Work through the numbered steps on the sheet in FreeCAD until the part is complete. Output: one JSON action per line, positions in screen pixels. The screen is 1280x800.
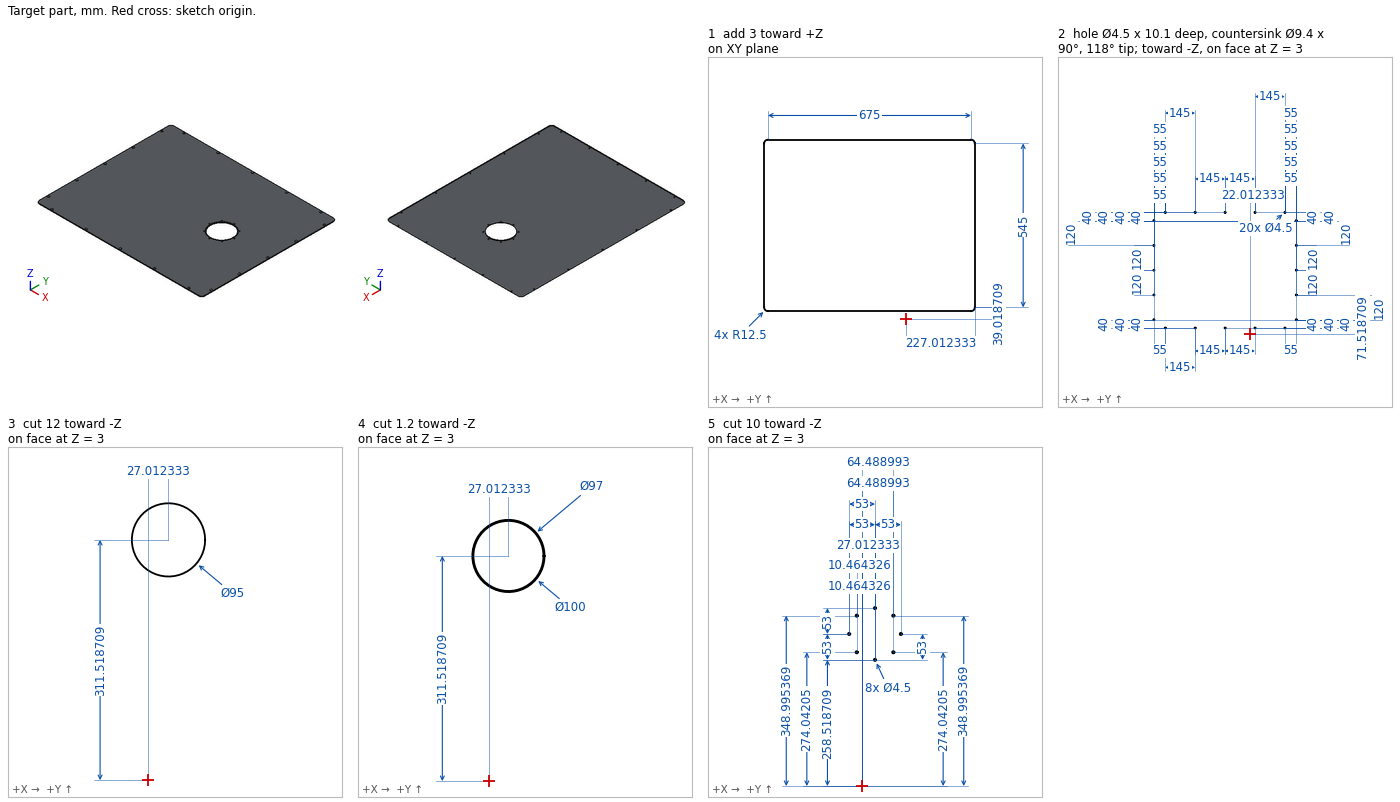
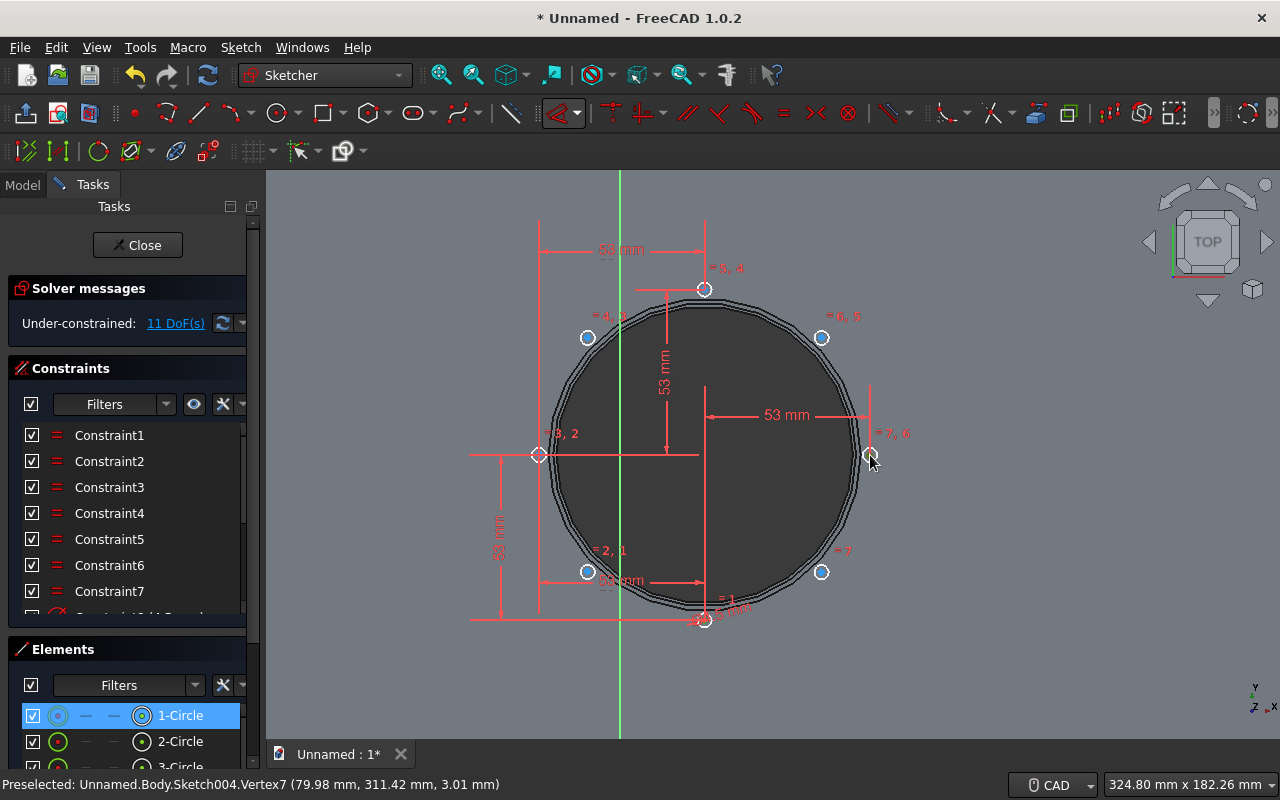
{"action": "left_click", "coordinate": [580, 114]}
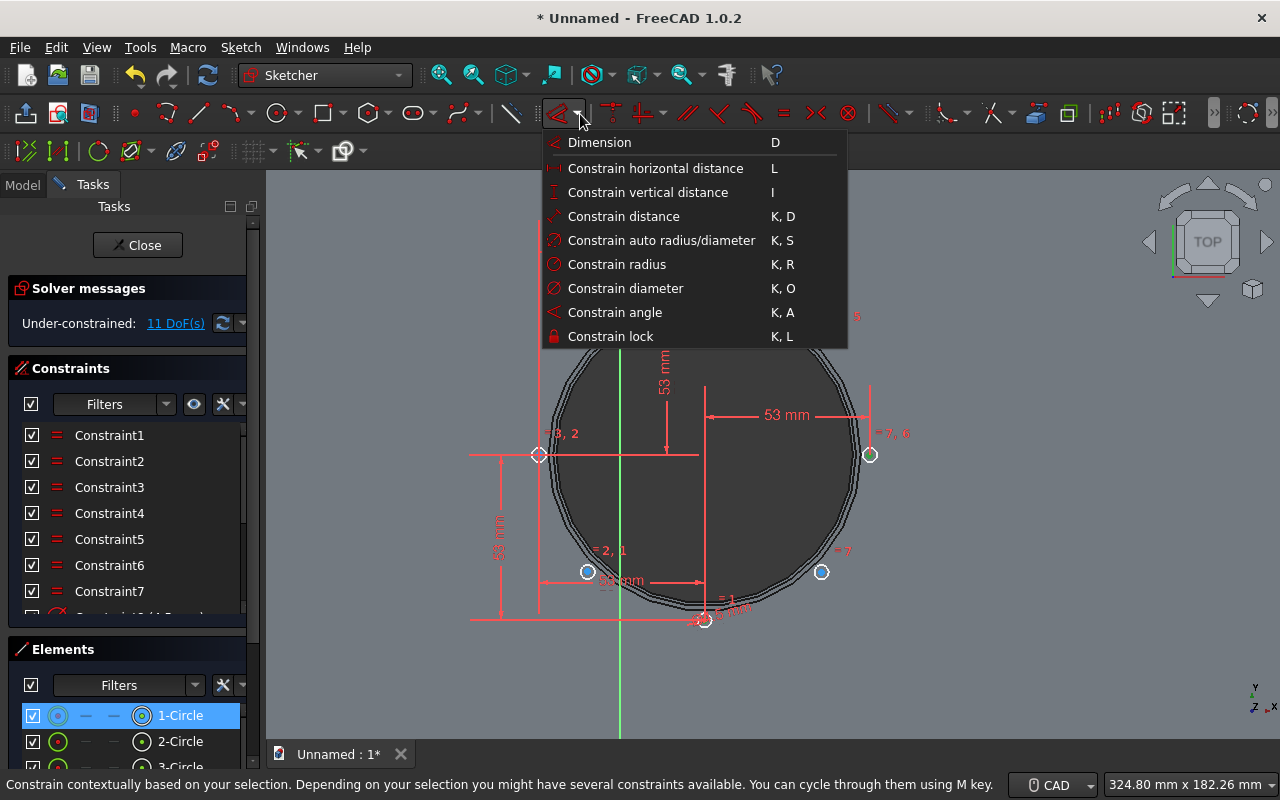
{"action": "left_click", "coordinate": [695, 192]}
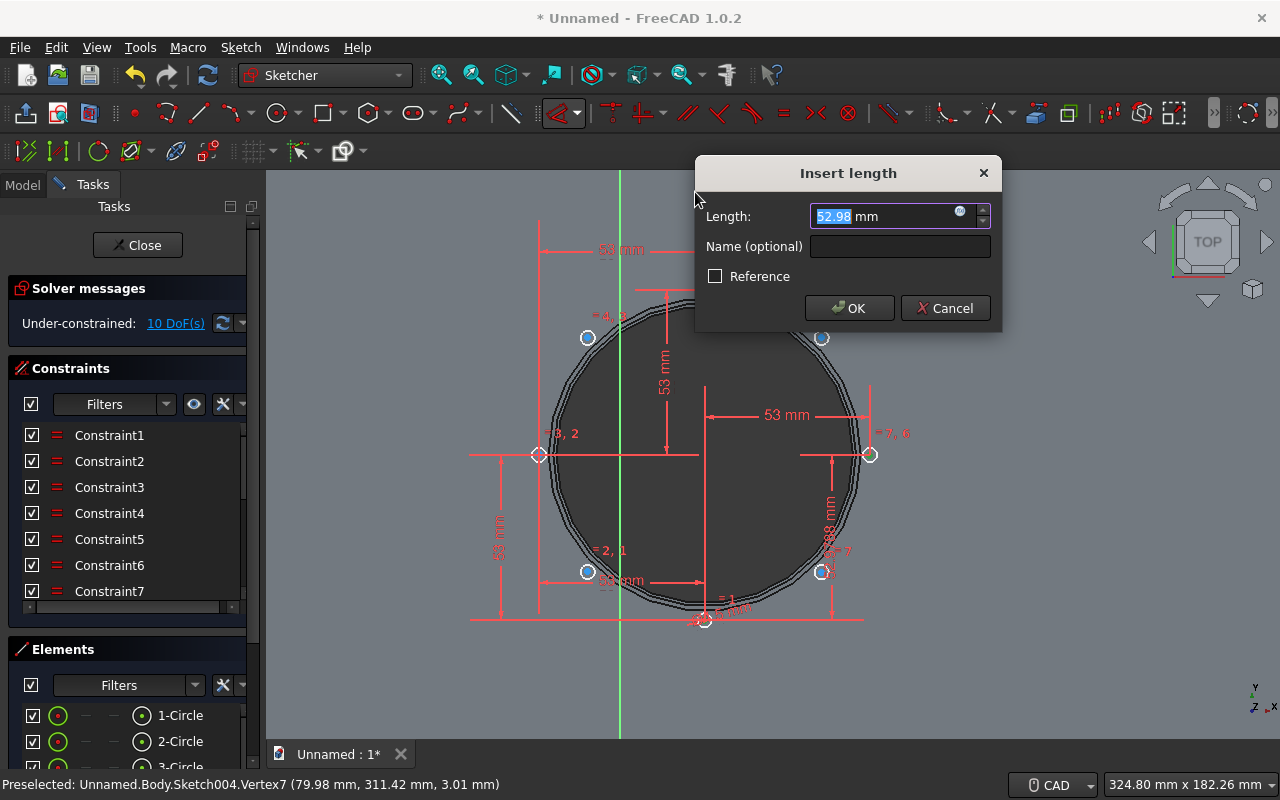
{"action": "type", "text": "53"}
{"action": "key", "text": "Return"}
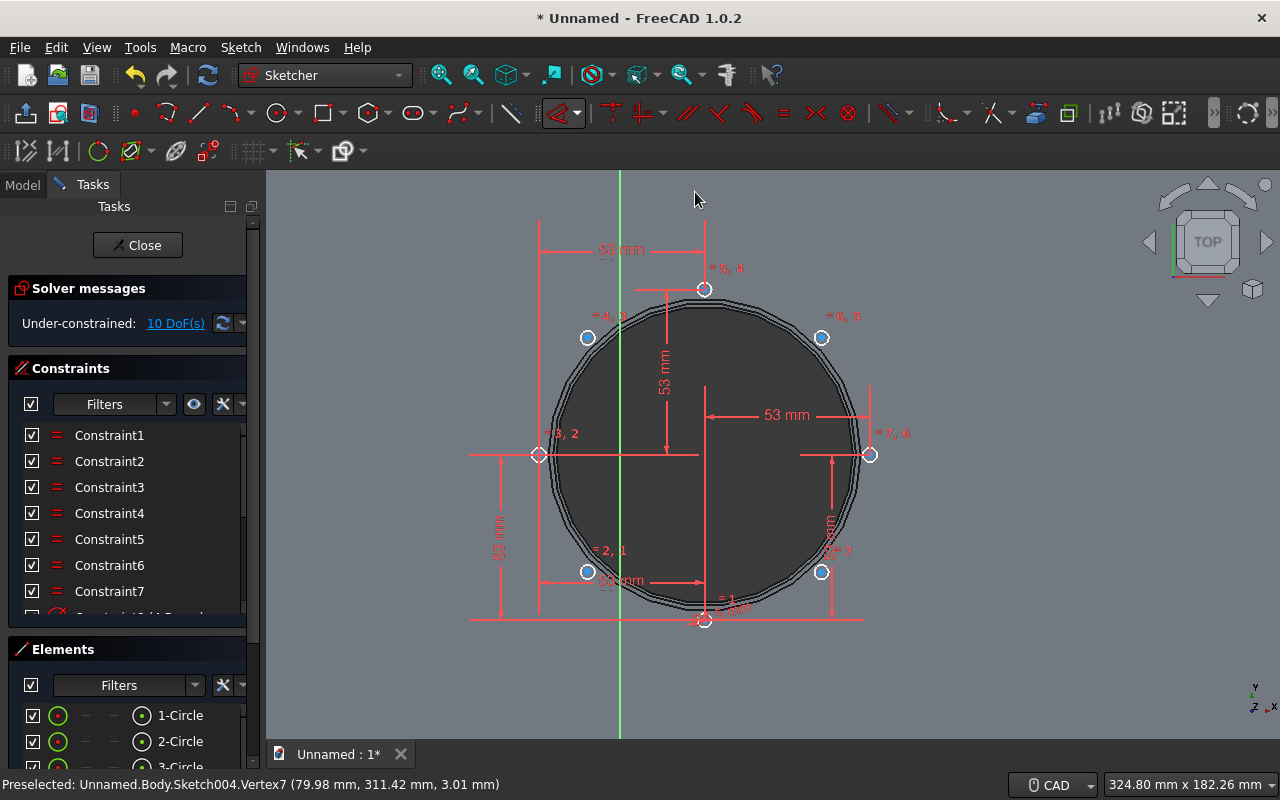
{"action": "left_click", "coordinate": [705, 620]}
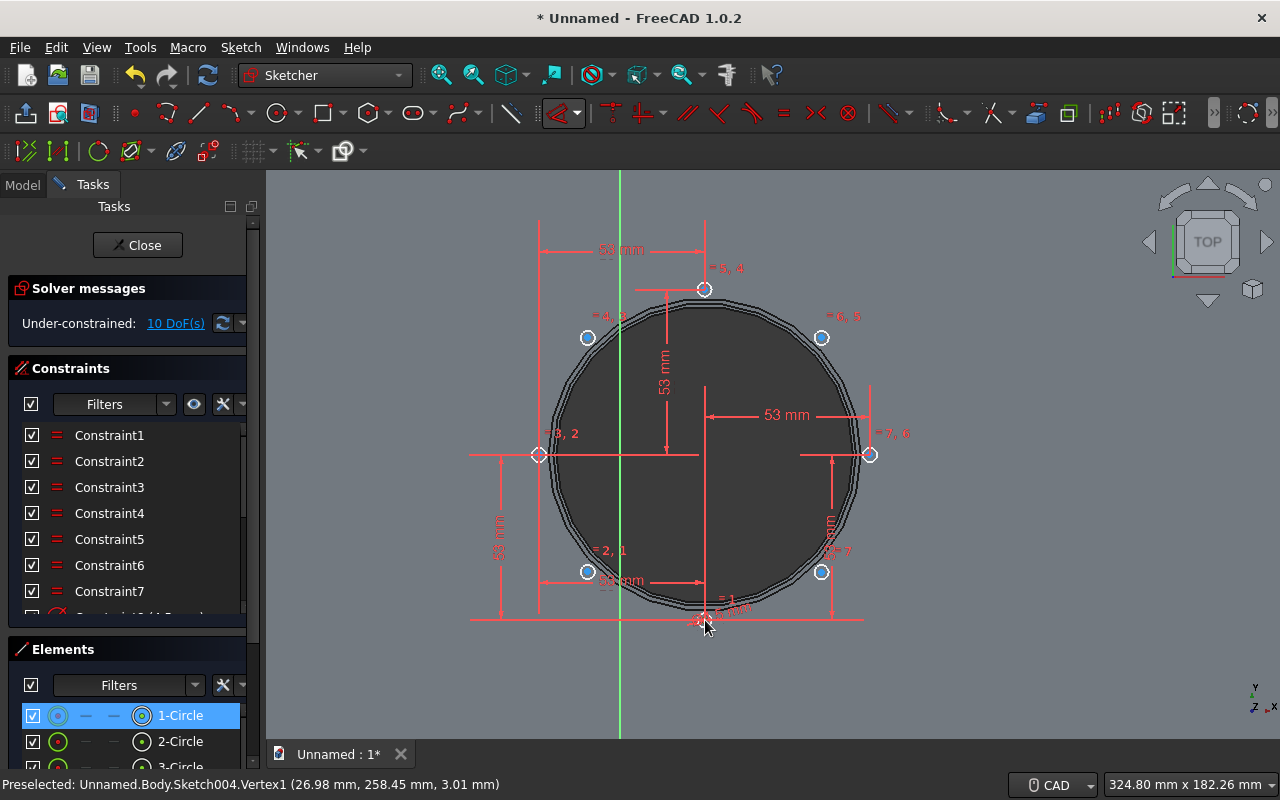
{"action": "left_click", "coordinate": [580, 114]}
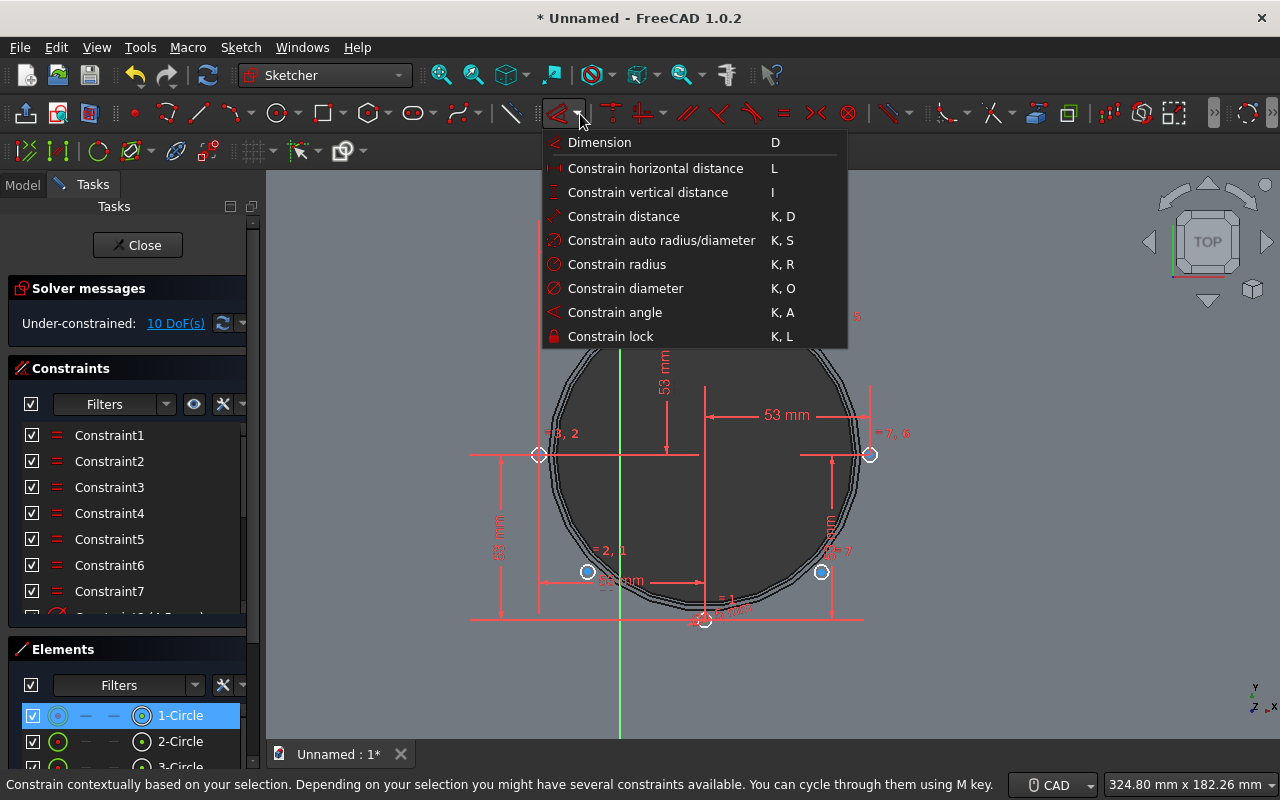
{"action": "left_click", "coordinate": [695, 168]}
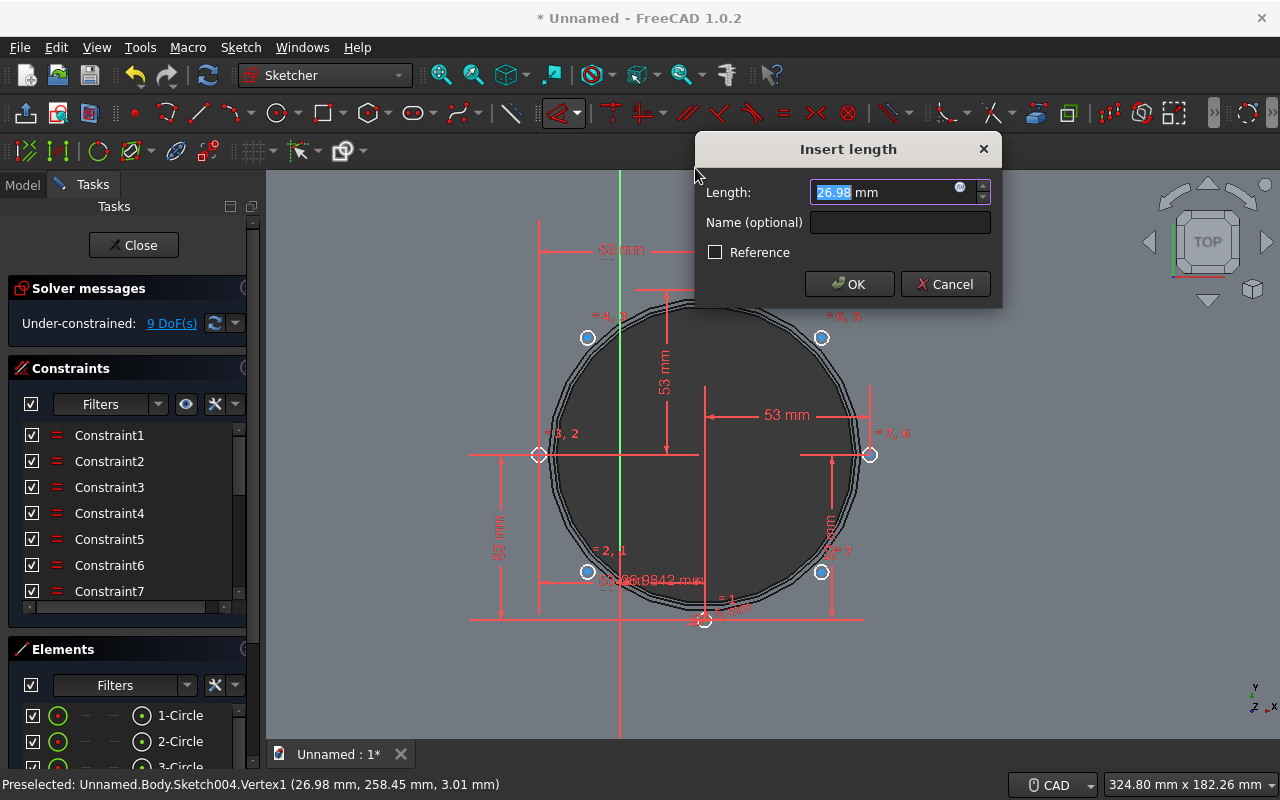
{"action": "type", "text": "27.012333"}
{"action": "key", "text": "Return"}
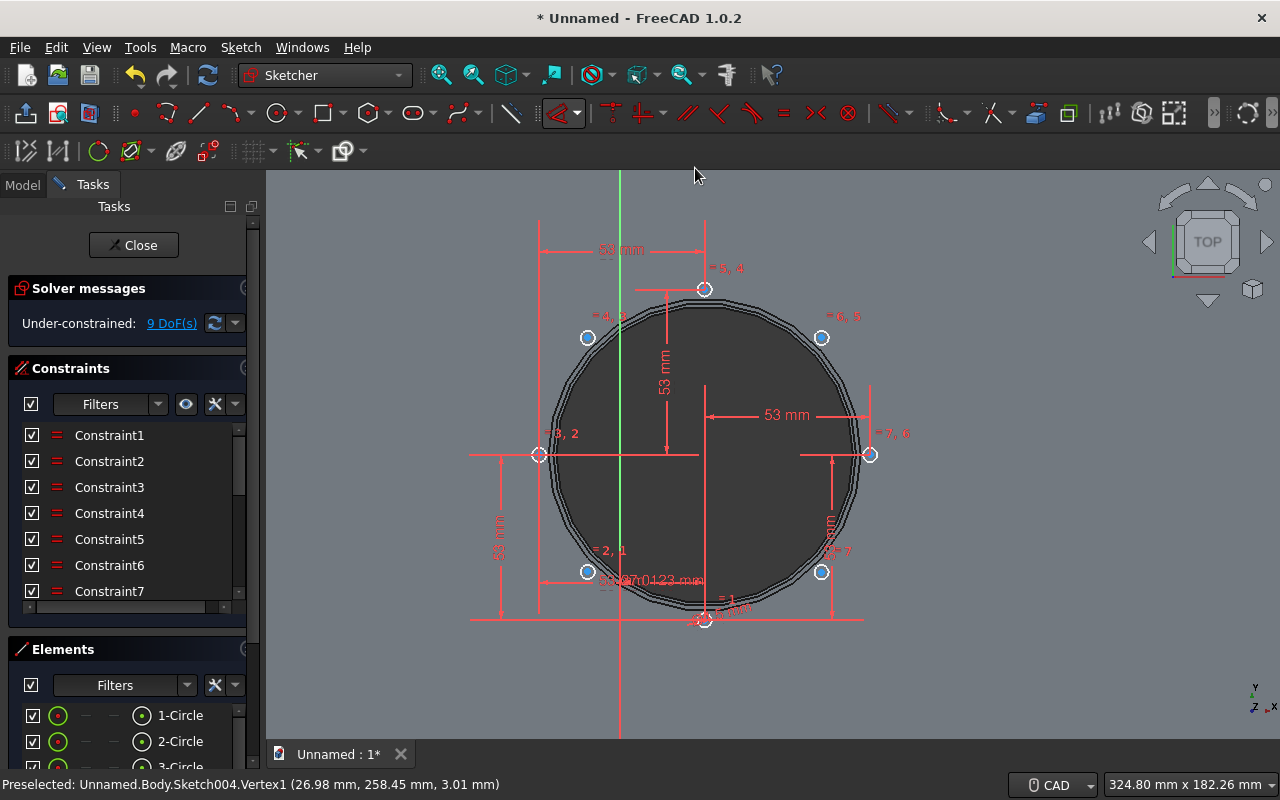
{"action": "left_click", "coordinate": [588, 572]}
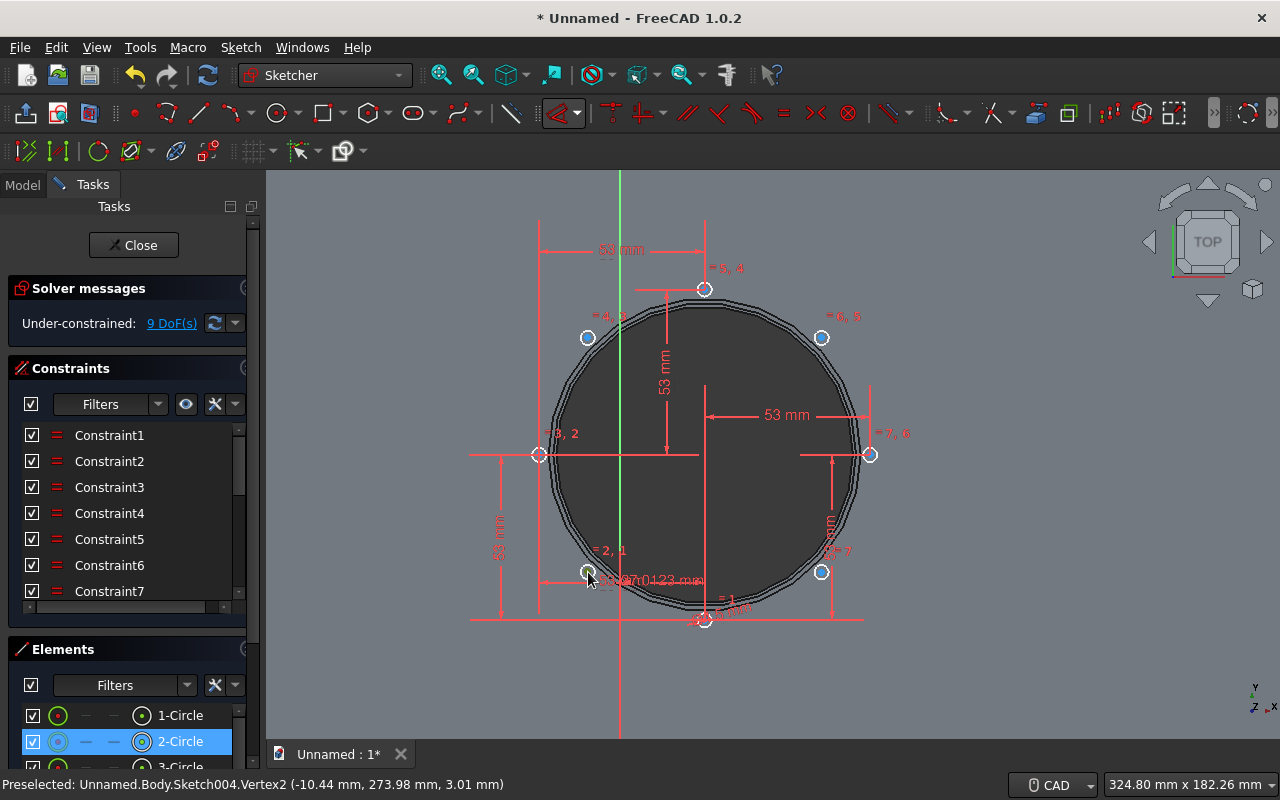
{"action": "left_click", "coordinate": [580, 114]}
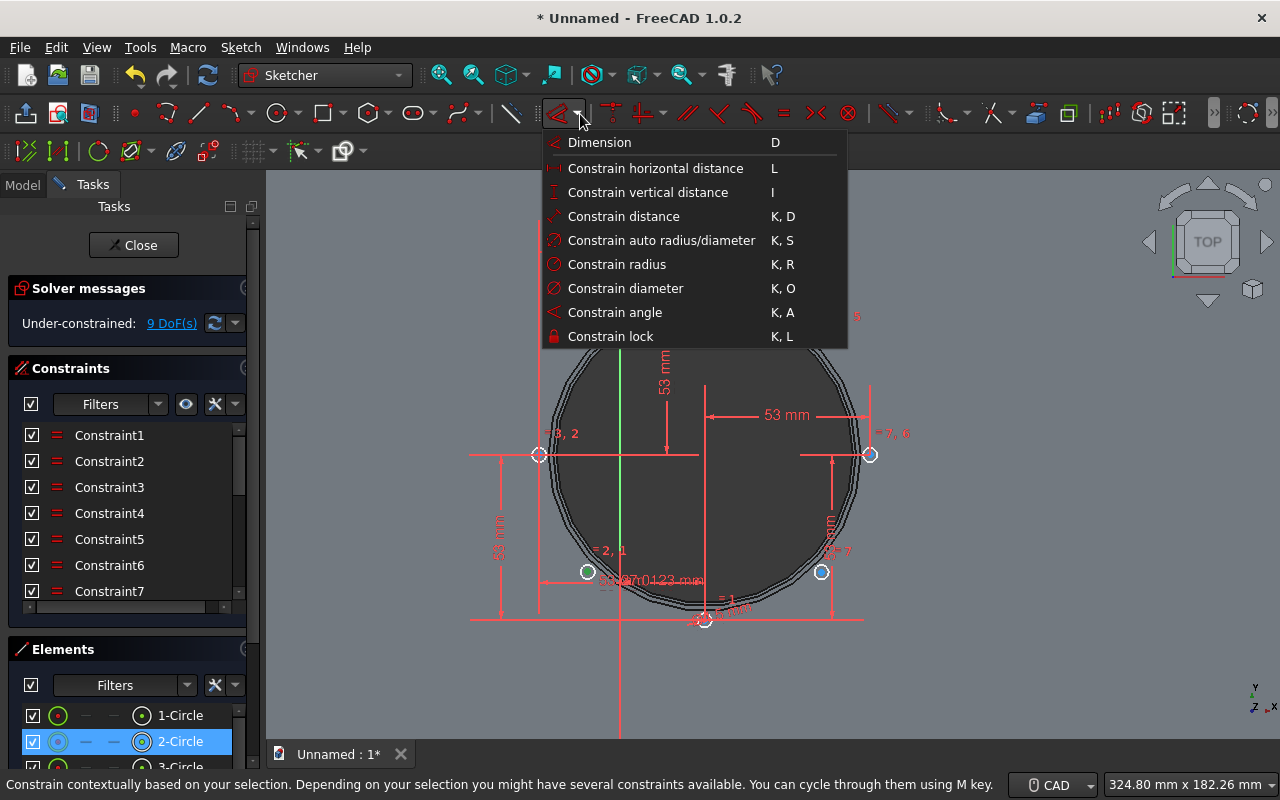
{"action": "left_click", "coordinate": [695, 168]}